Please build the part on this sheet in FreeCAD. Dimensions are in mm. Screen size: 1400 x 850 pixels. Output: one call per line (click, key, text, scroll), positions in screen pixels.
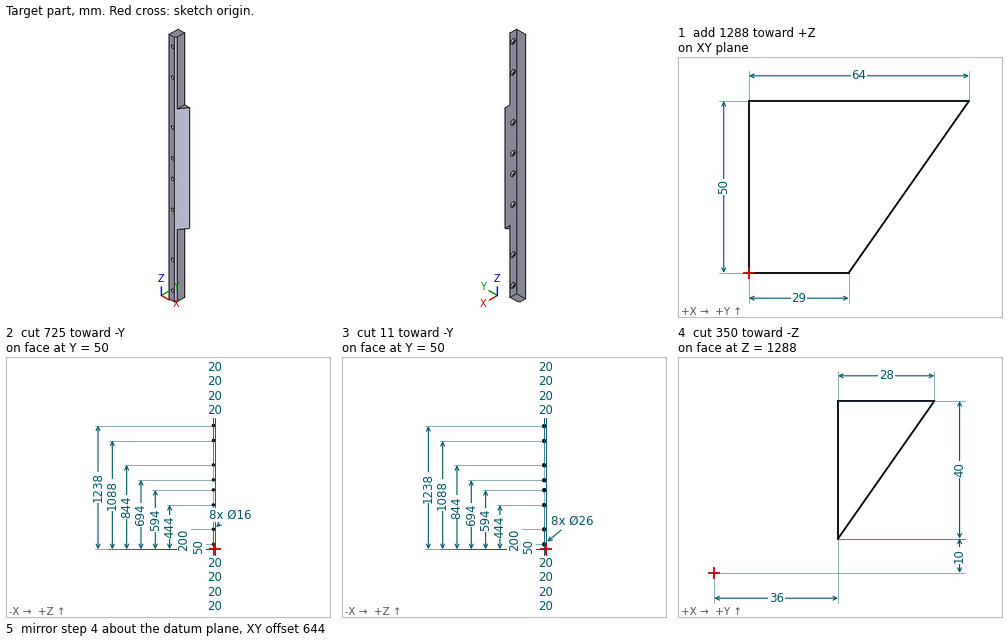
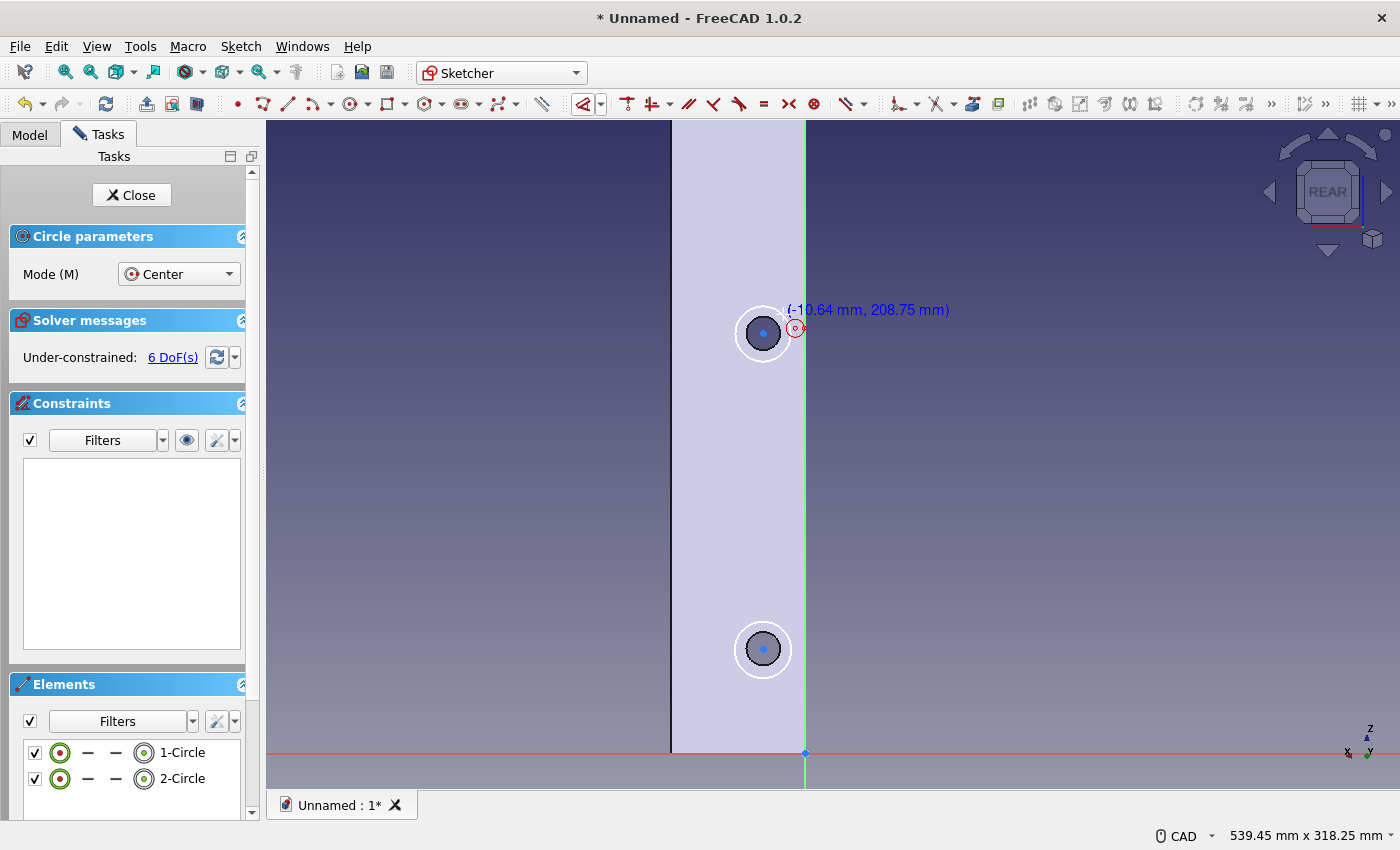
scroll(763, 656, down, 9)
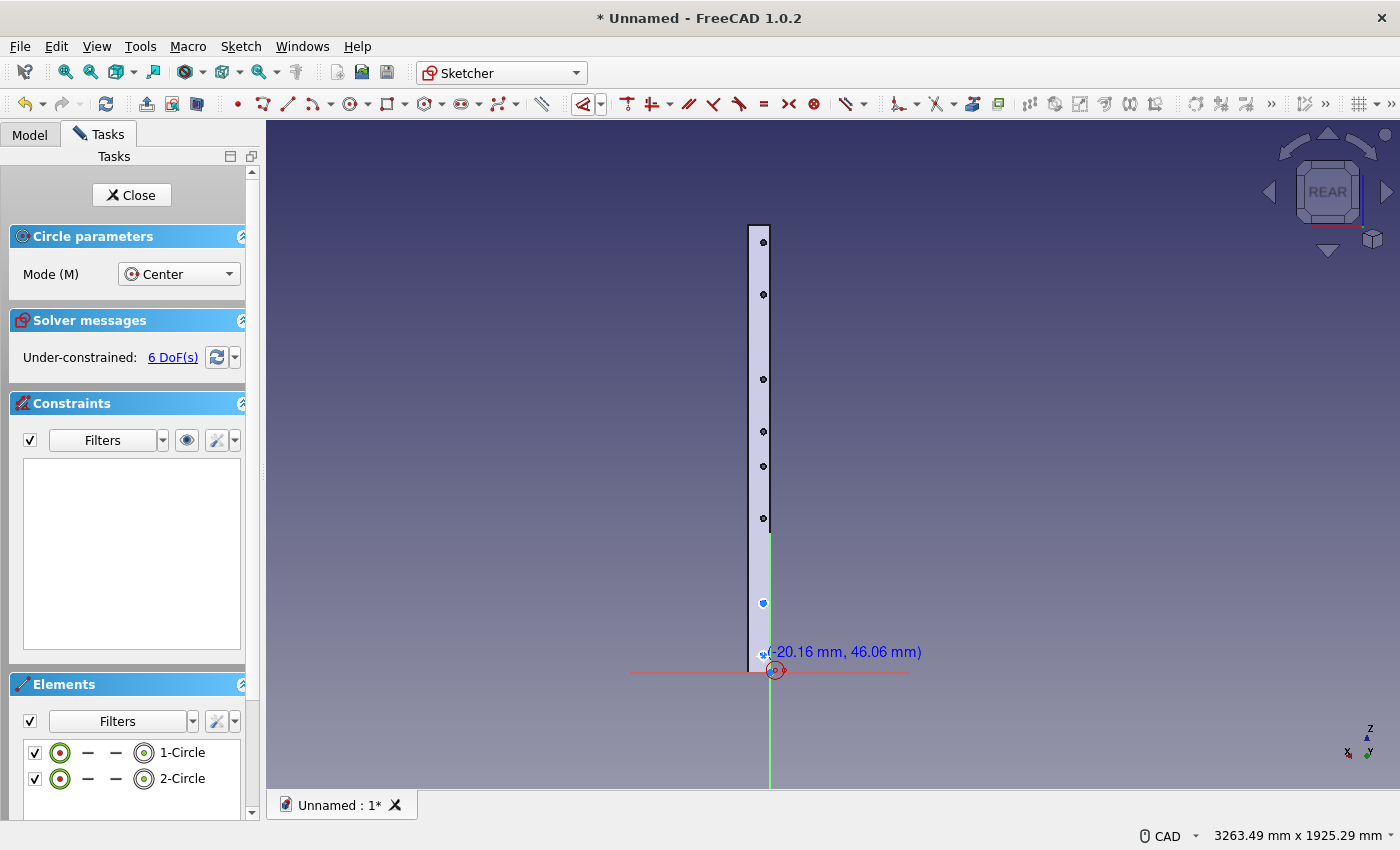
scroll(763, 519, up, 9)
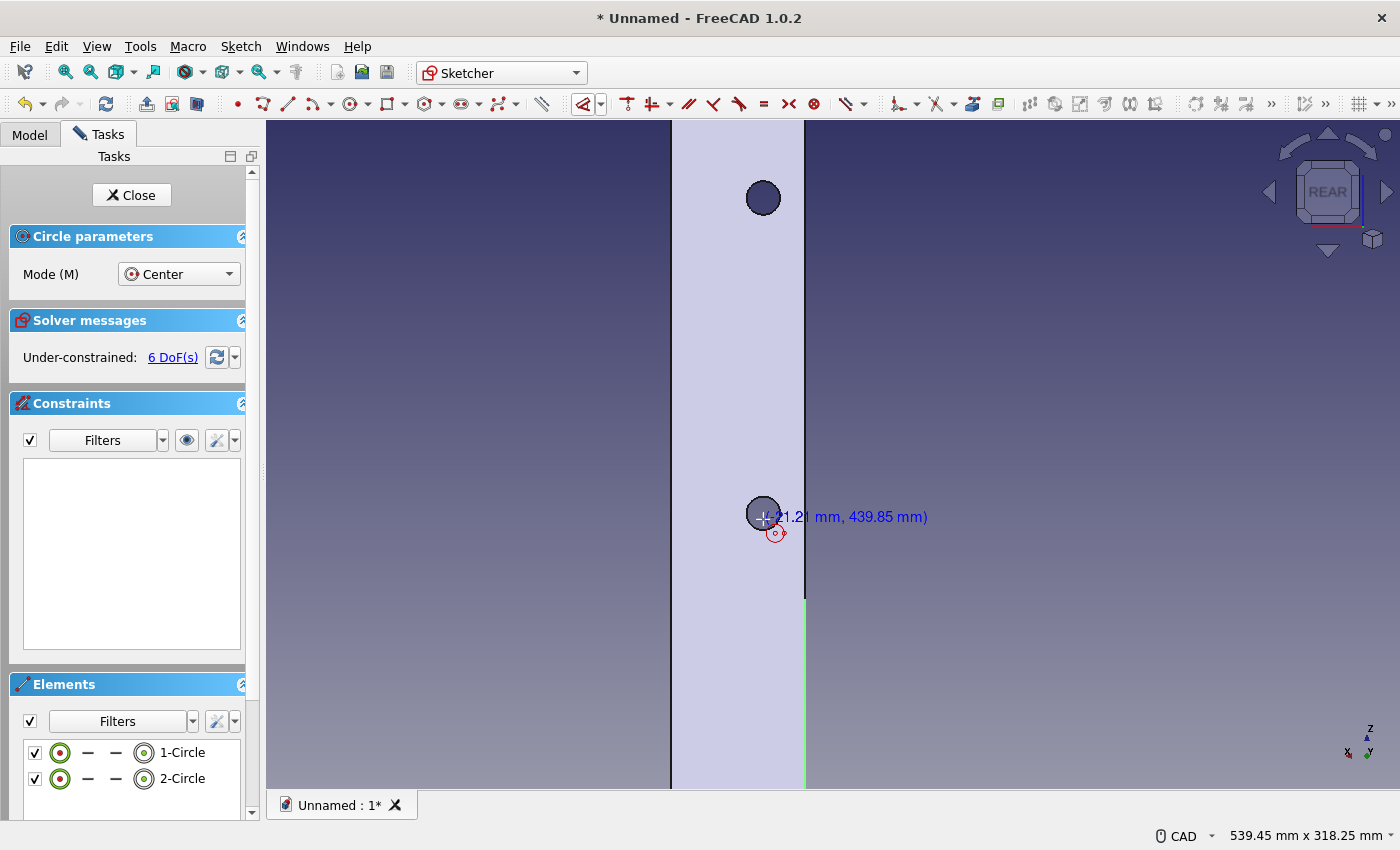
click(763, 513)
click(783, 494)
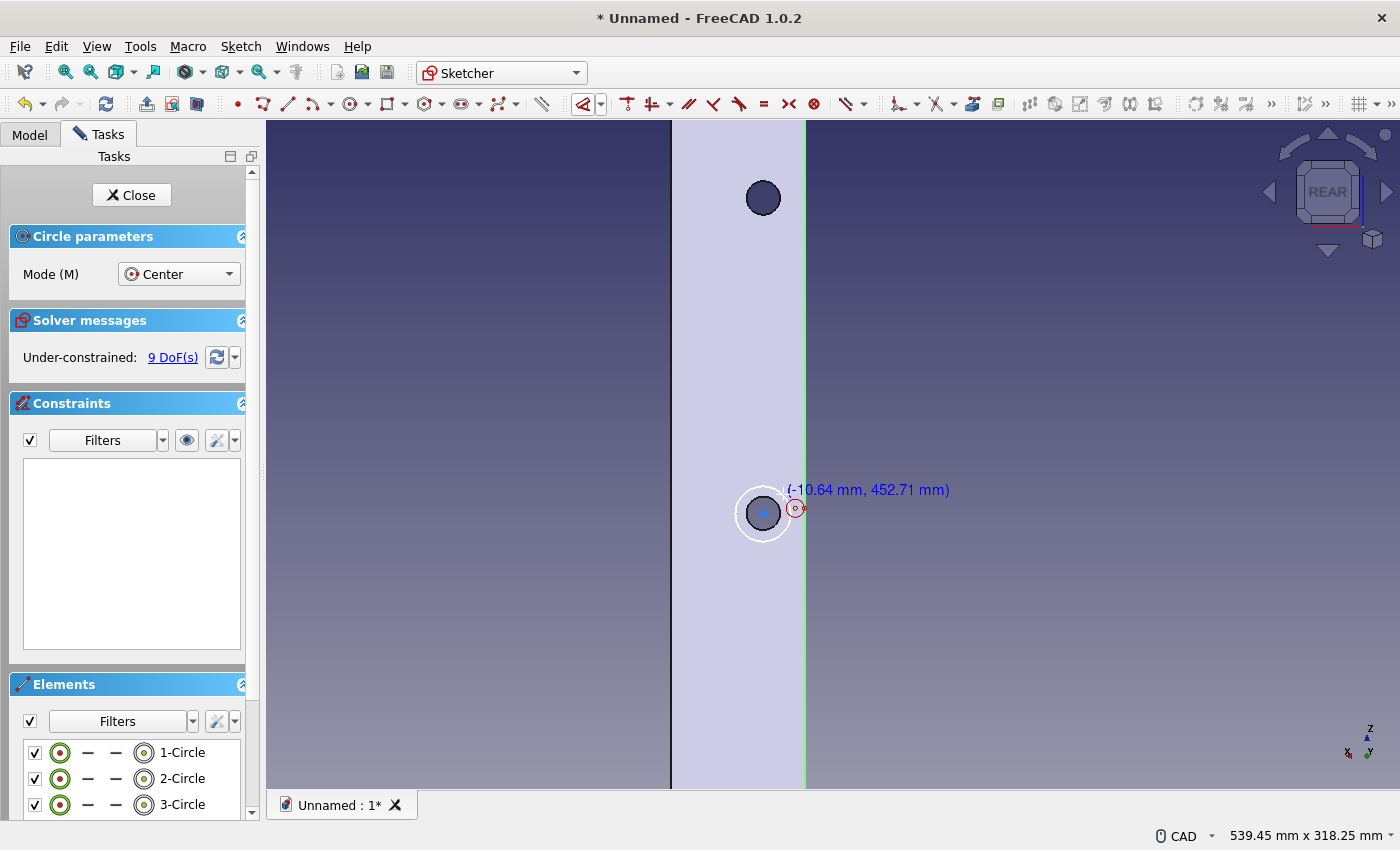
click(763, 198)
click(783, 179)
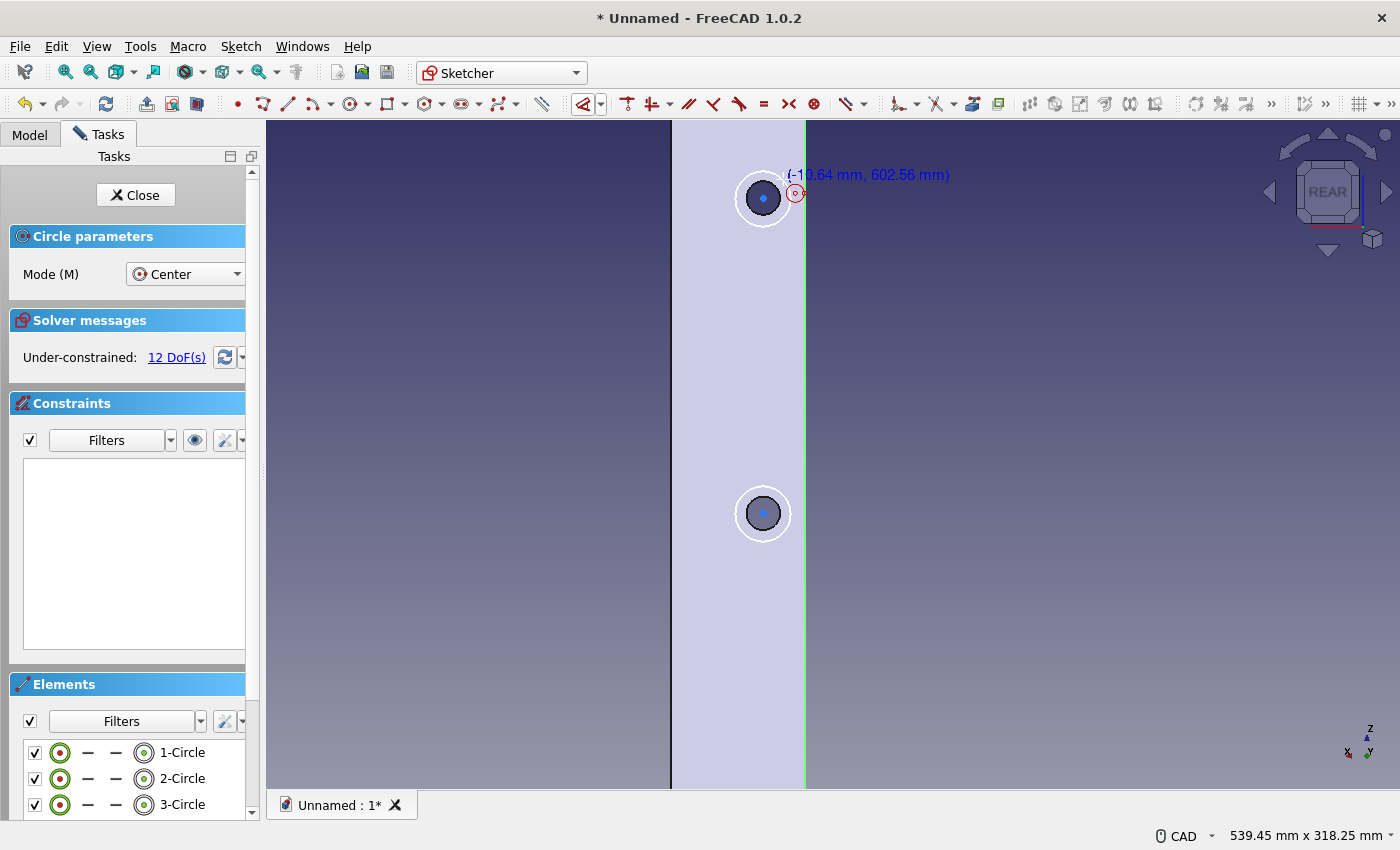
scroll(763, 518, down, 9)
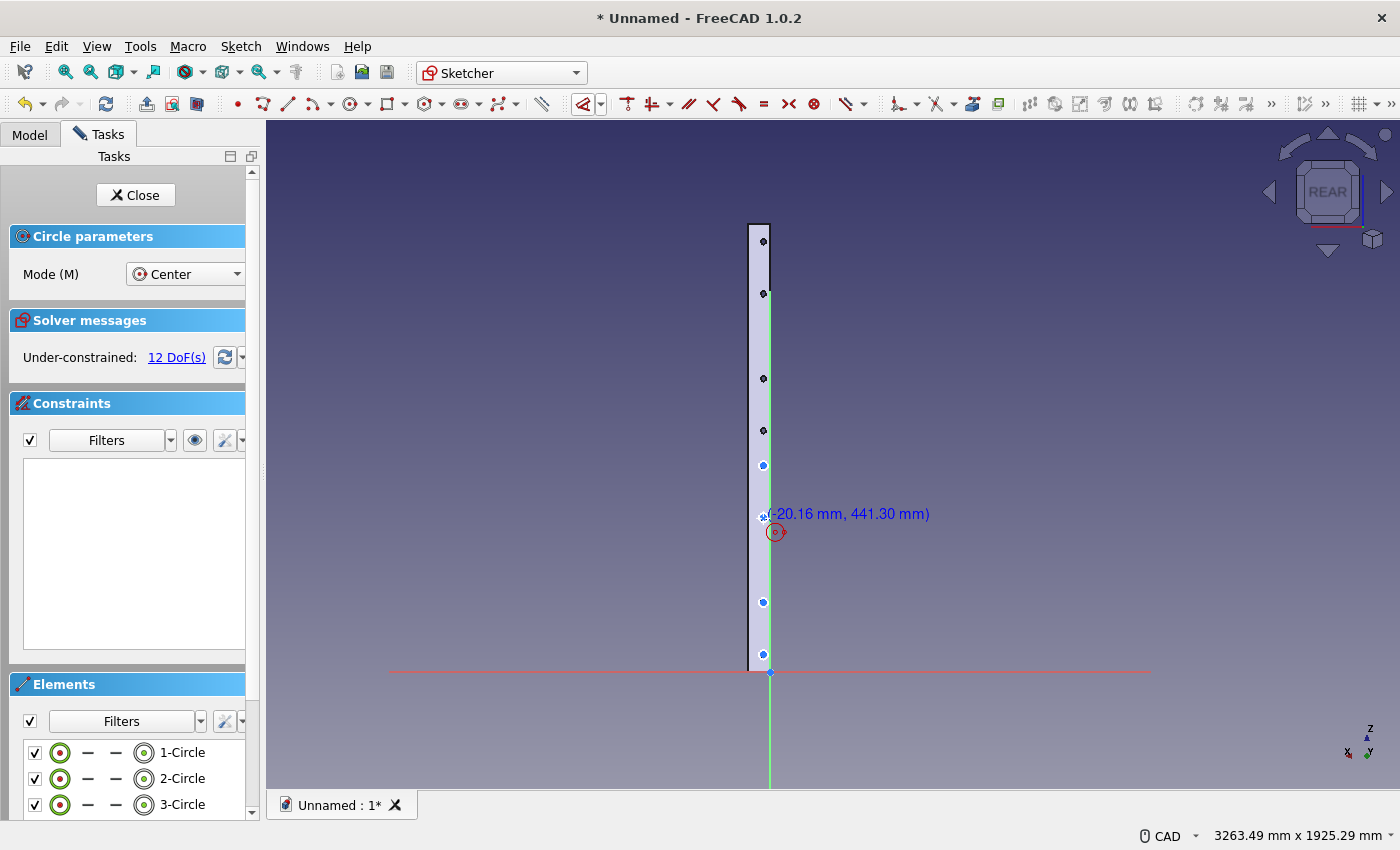
scroll(763, 431, up, 9)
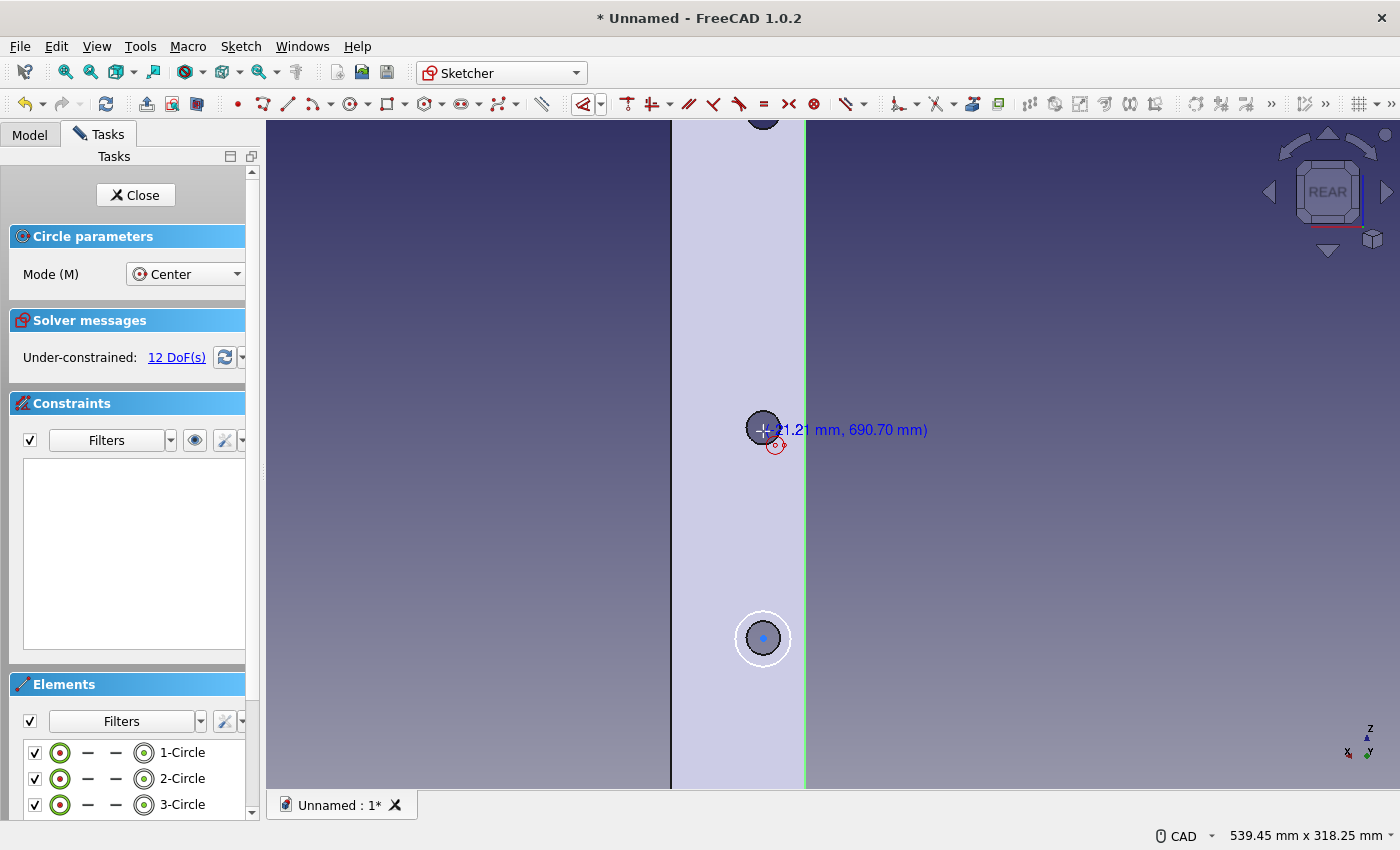
click(763, 428)
click(783, 408)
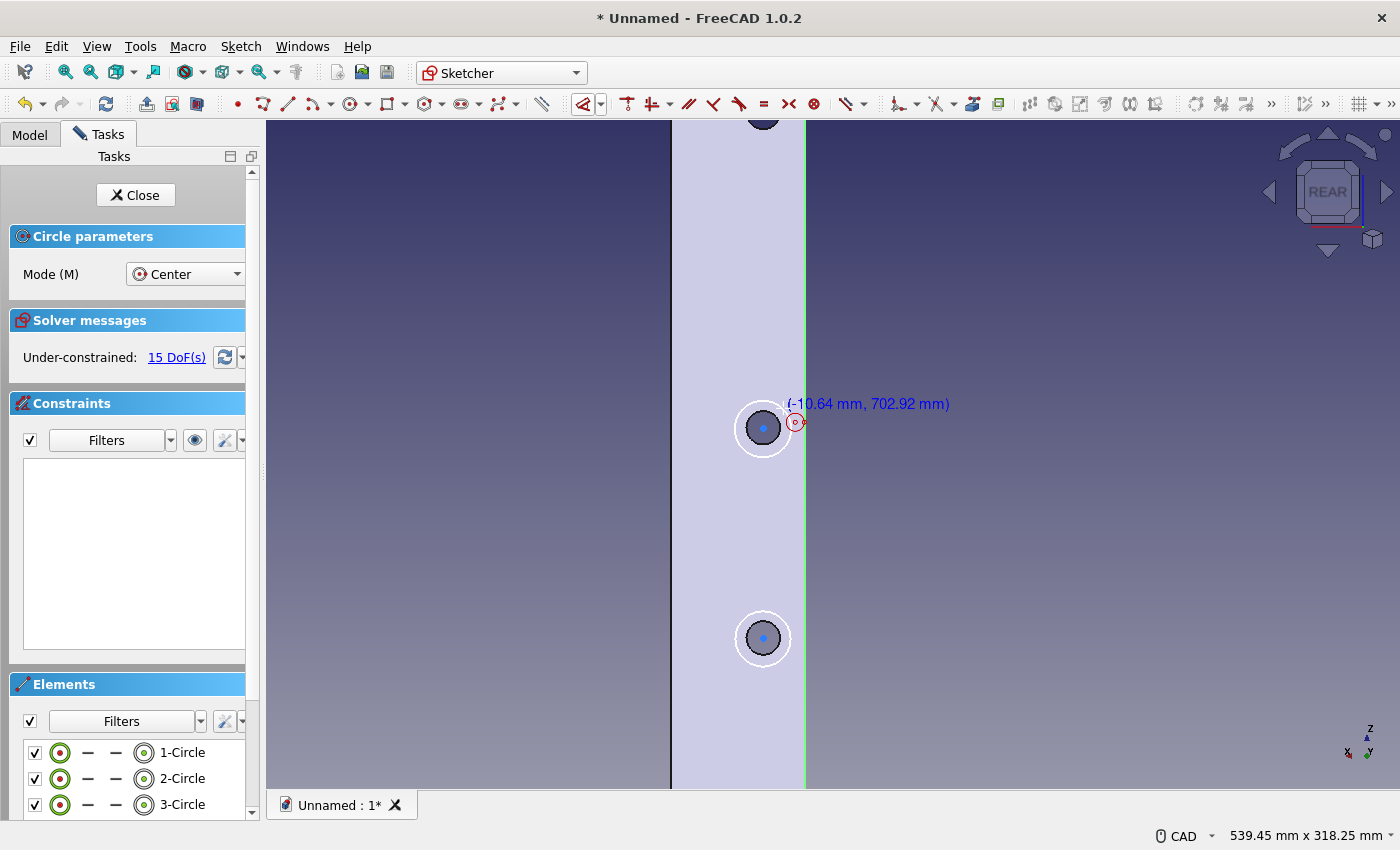
scroll(763, 431, down, 9)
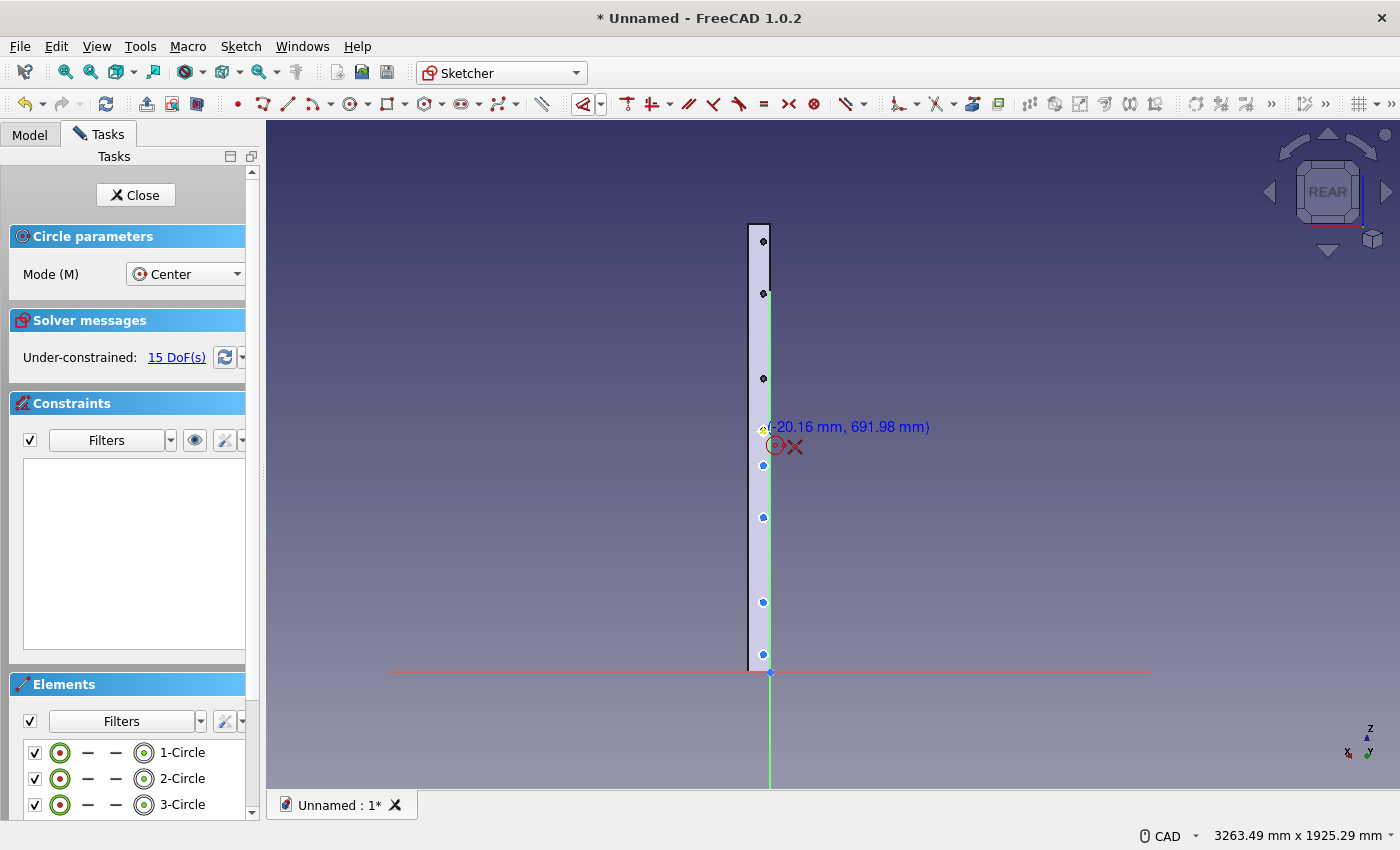
scroll(763, 379, up, 9)